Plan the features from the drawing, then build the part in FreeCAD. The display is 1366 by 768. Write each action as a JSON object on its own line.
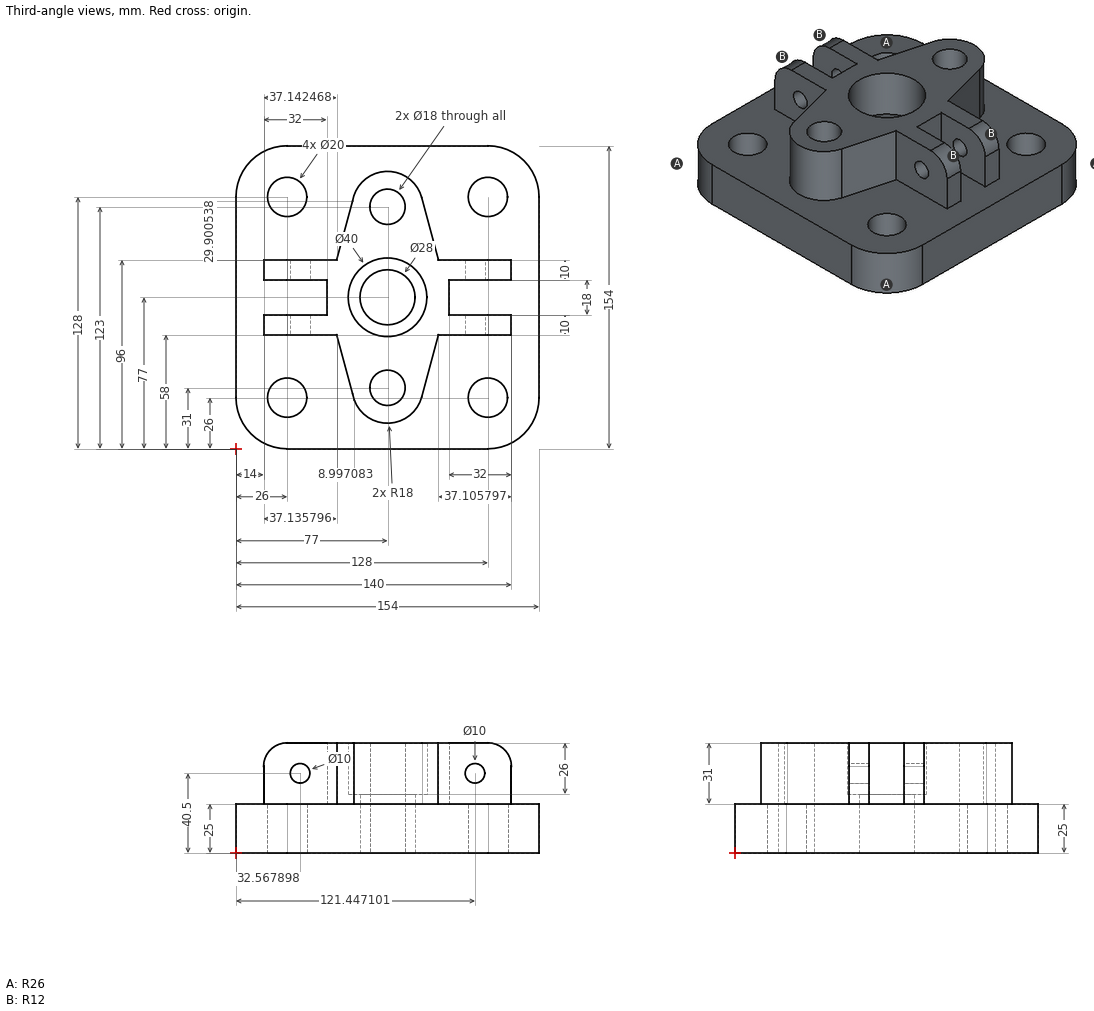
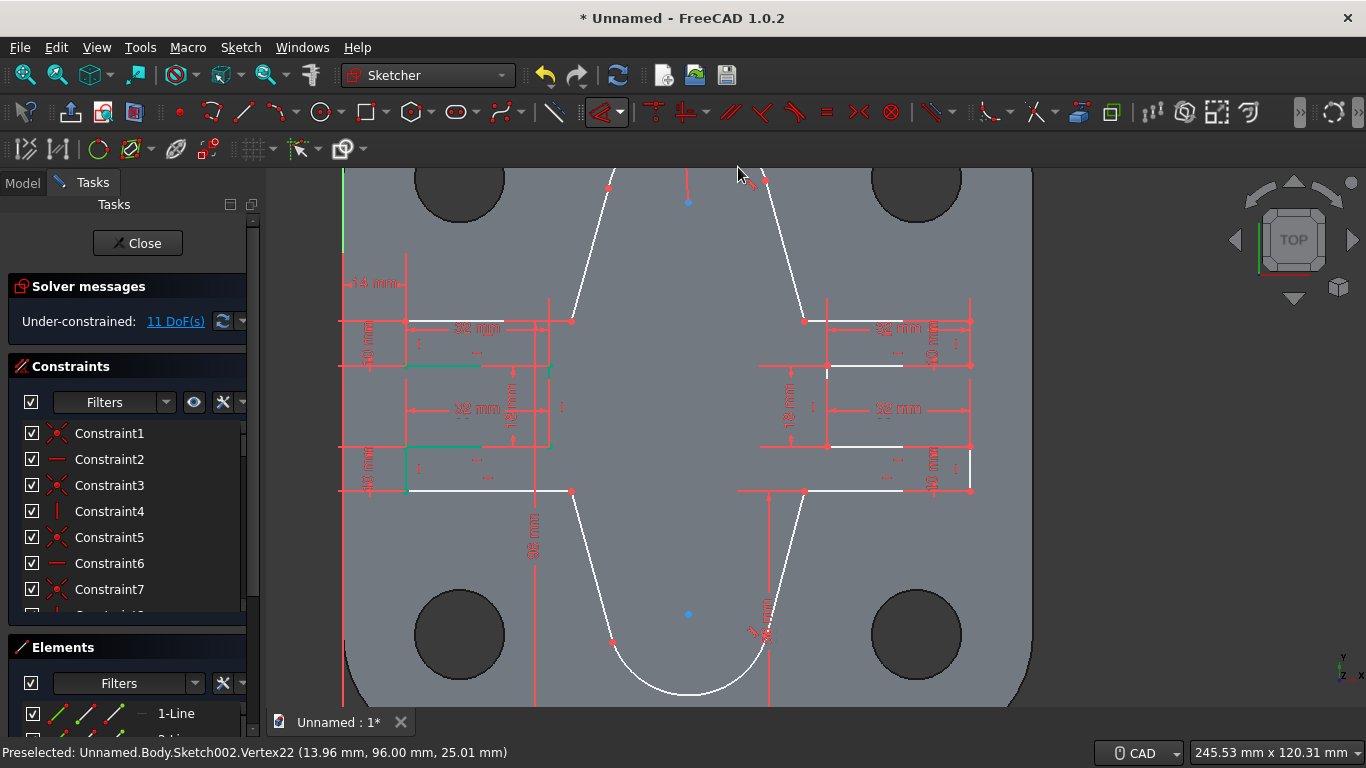
{"action": "left_click", "coordinate": [688, 202]}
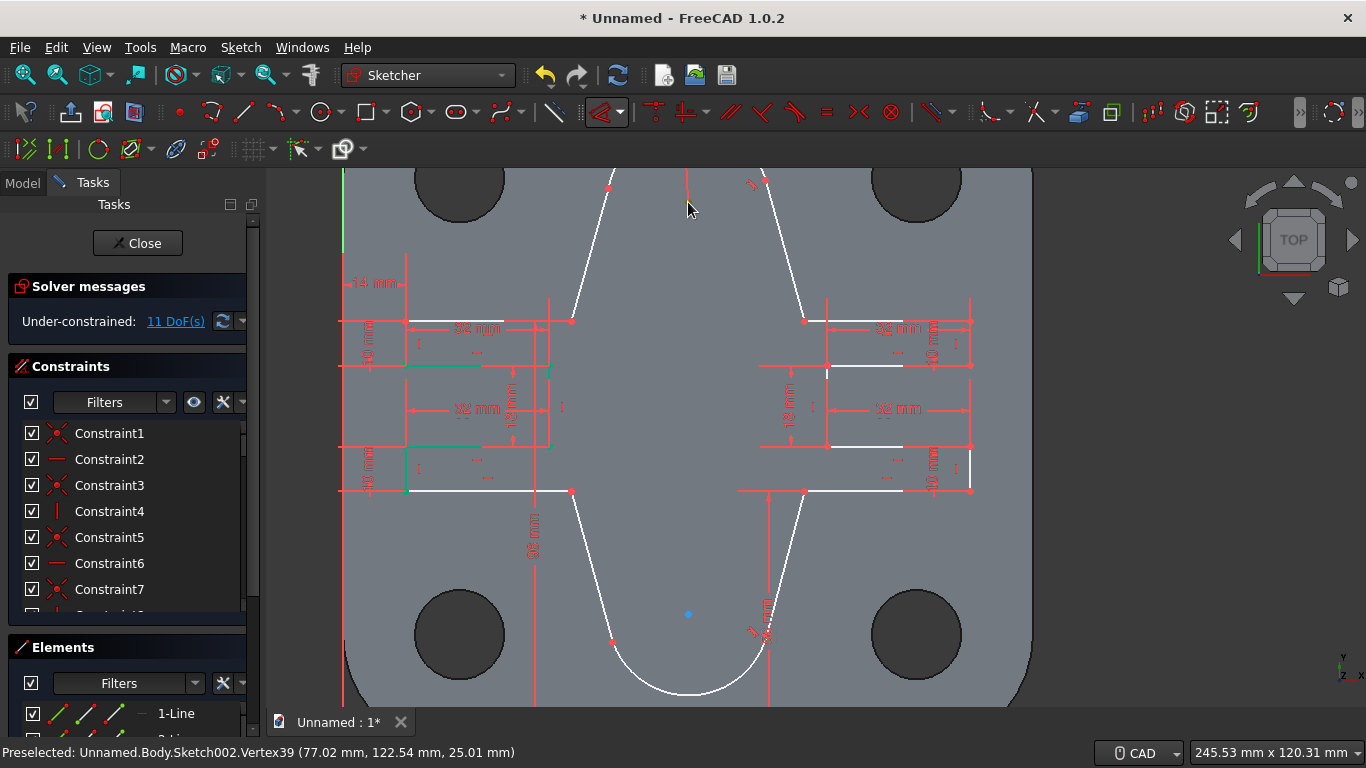
{"action": "left_click", "coordinate": [622, 112]}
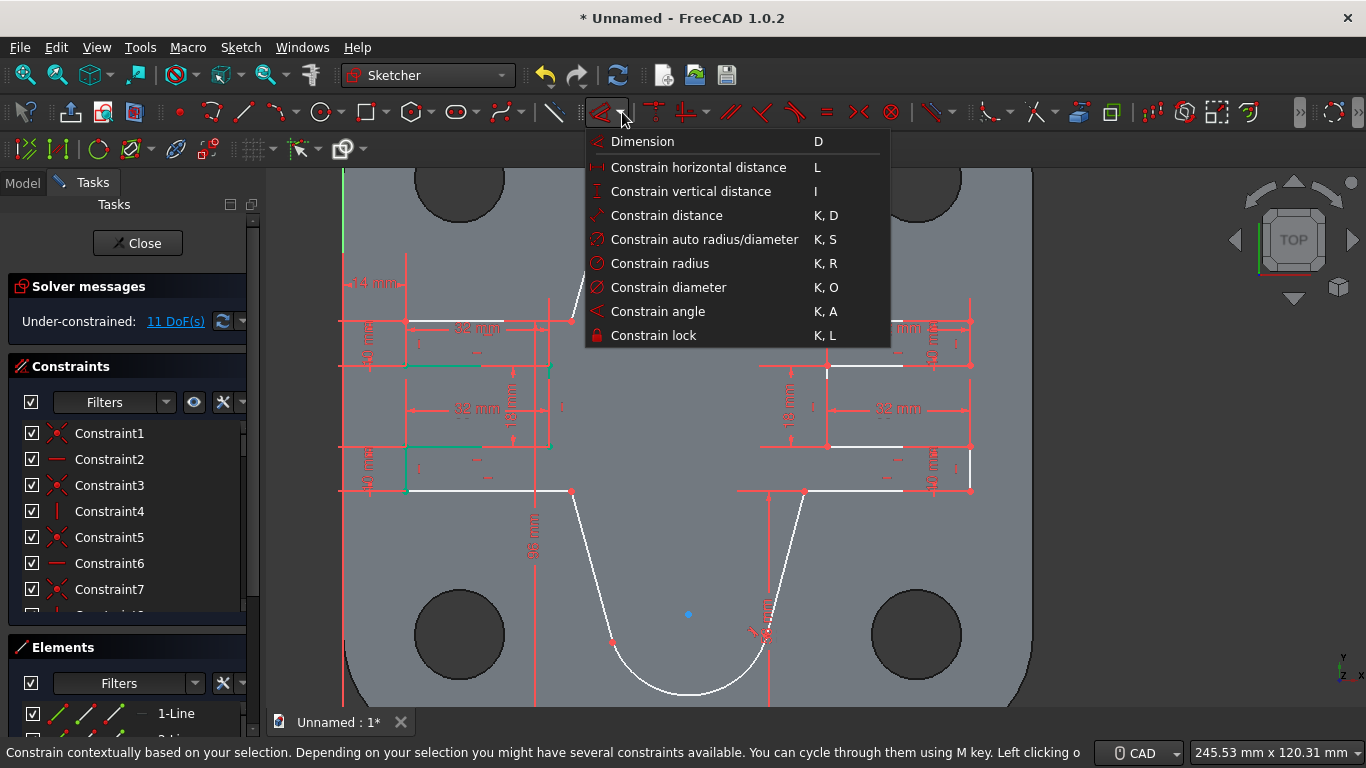
{"action": "left_click", "coordinate": [738, 167]}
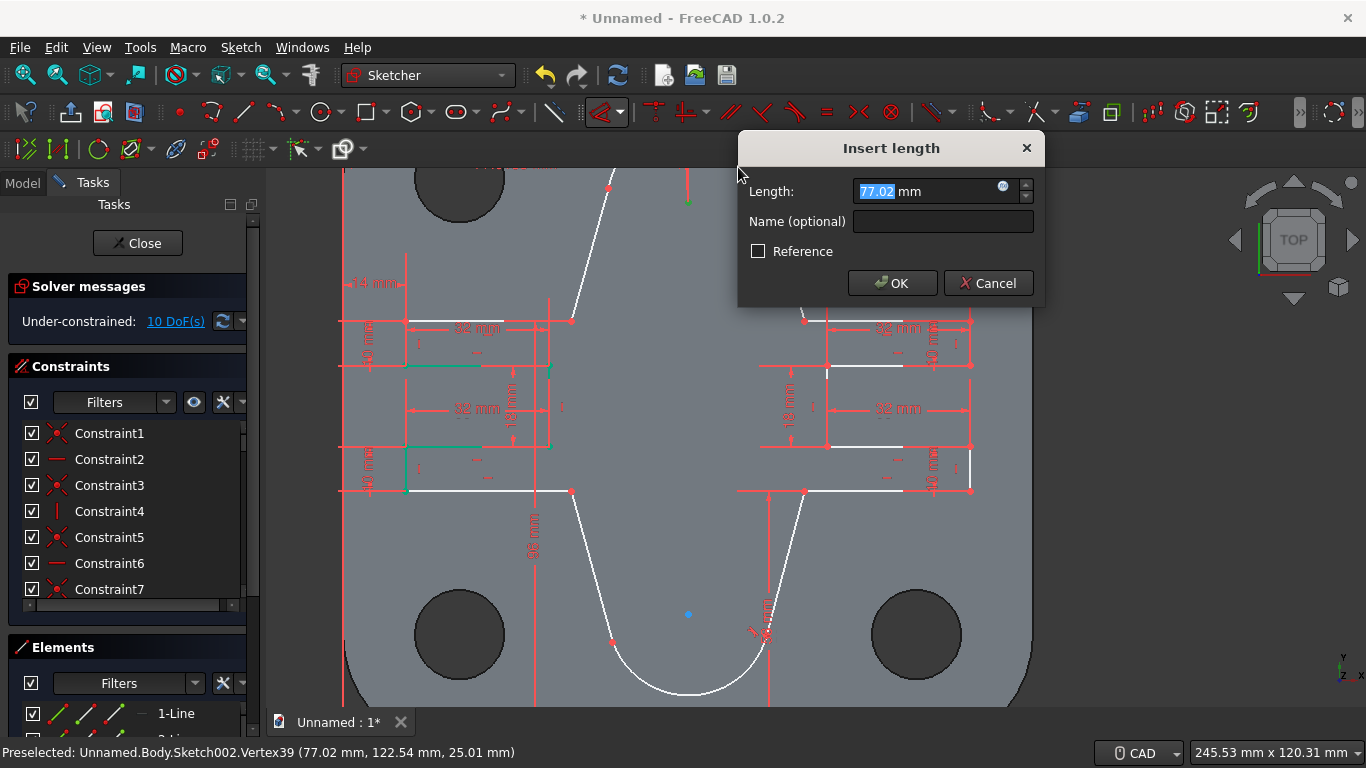
{"action": "type", "text": "77"}
{"action": "key", "text": "Return"}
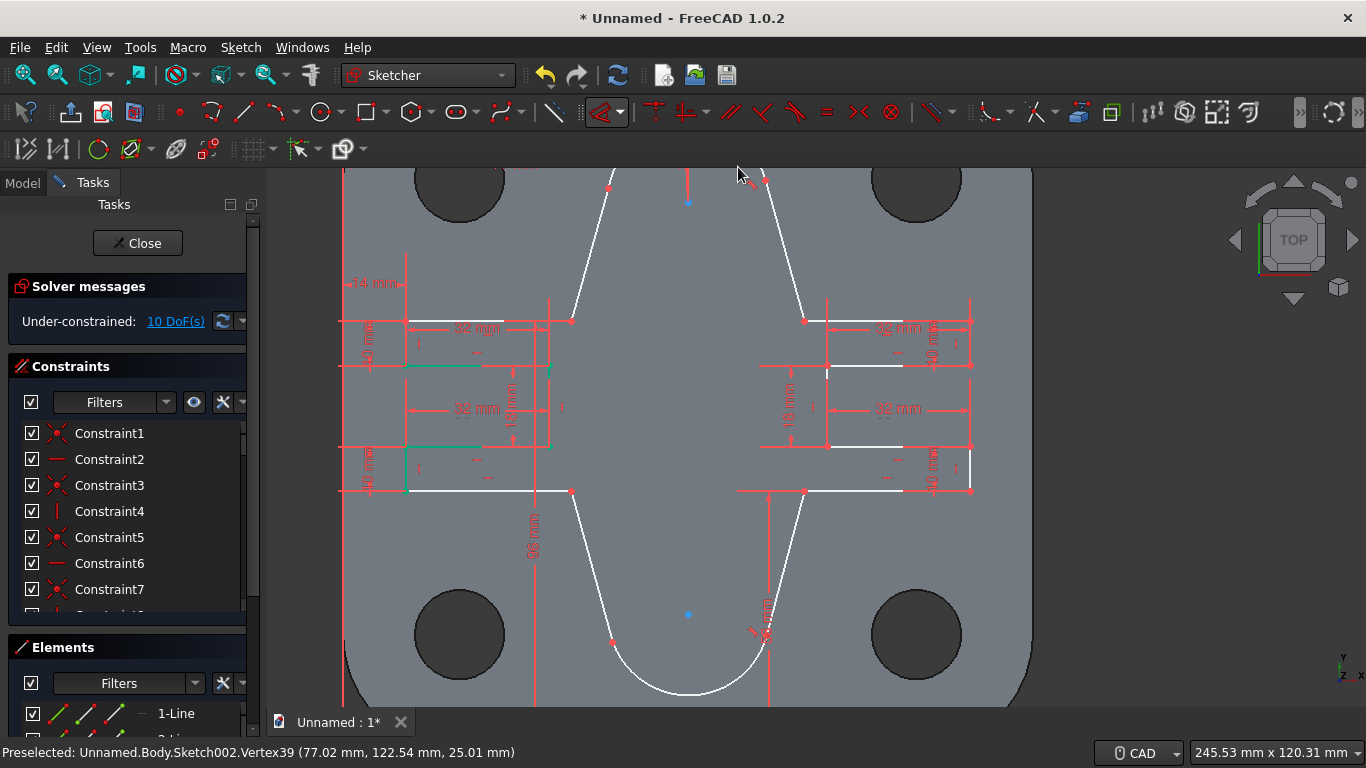
{"action": "left_click", "coordinate": [689, 615]}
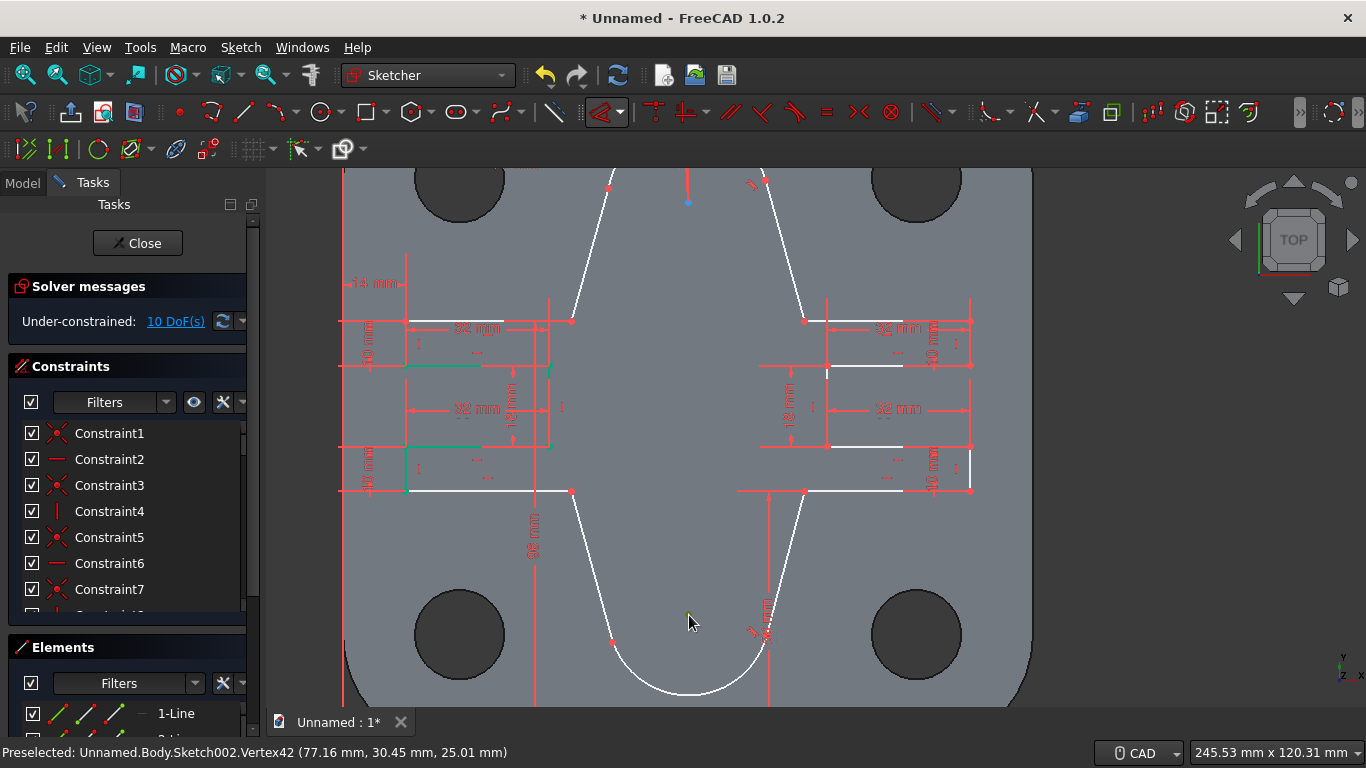
{"action": "left_click", "coordinate": [622, 112]}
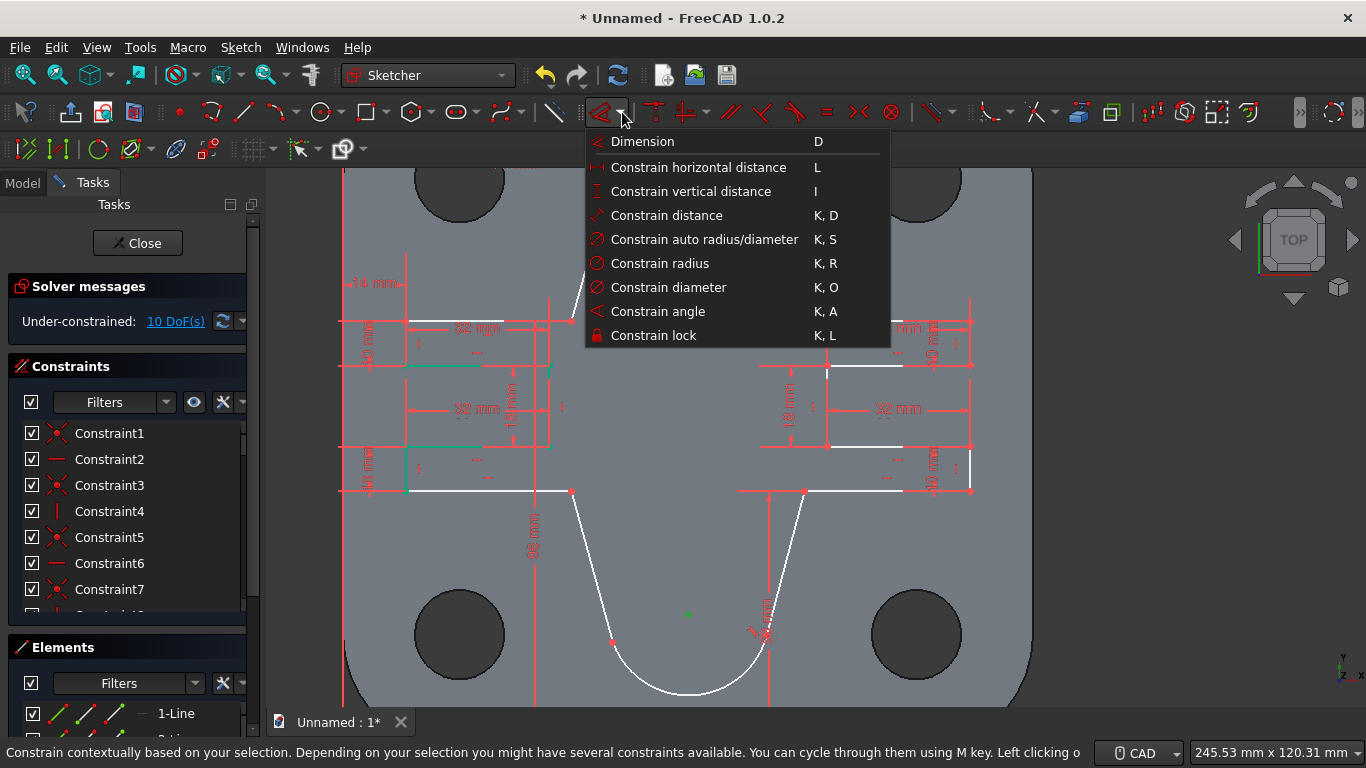
{"action": "left_click", "coordinate": [738, 167]}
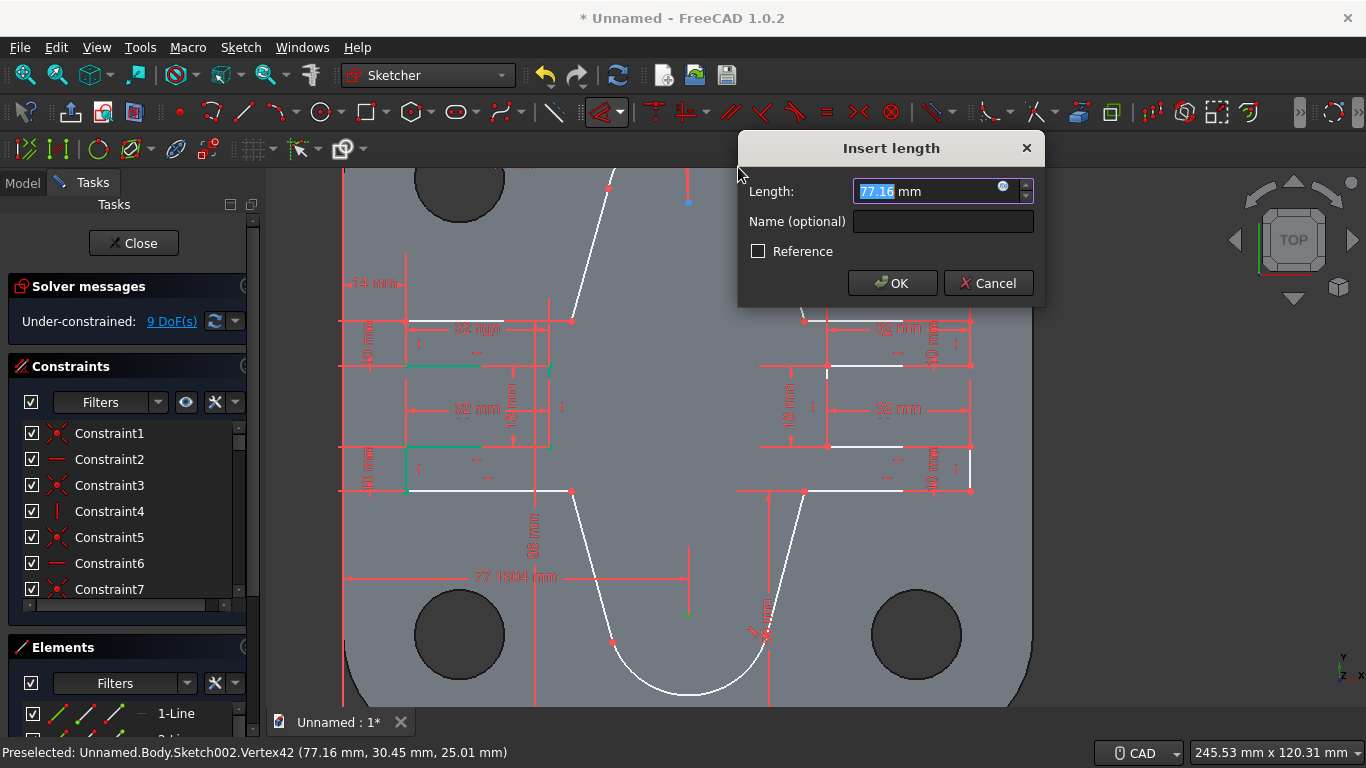
{"action": "type", "text": "77"}
{"action": "key", "text": "Return"}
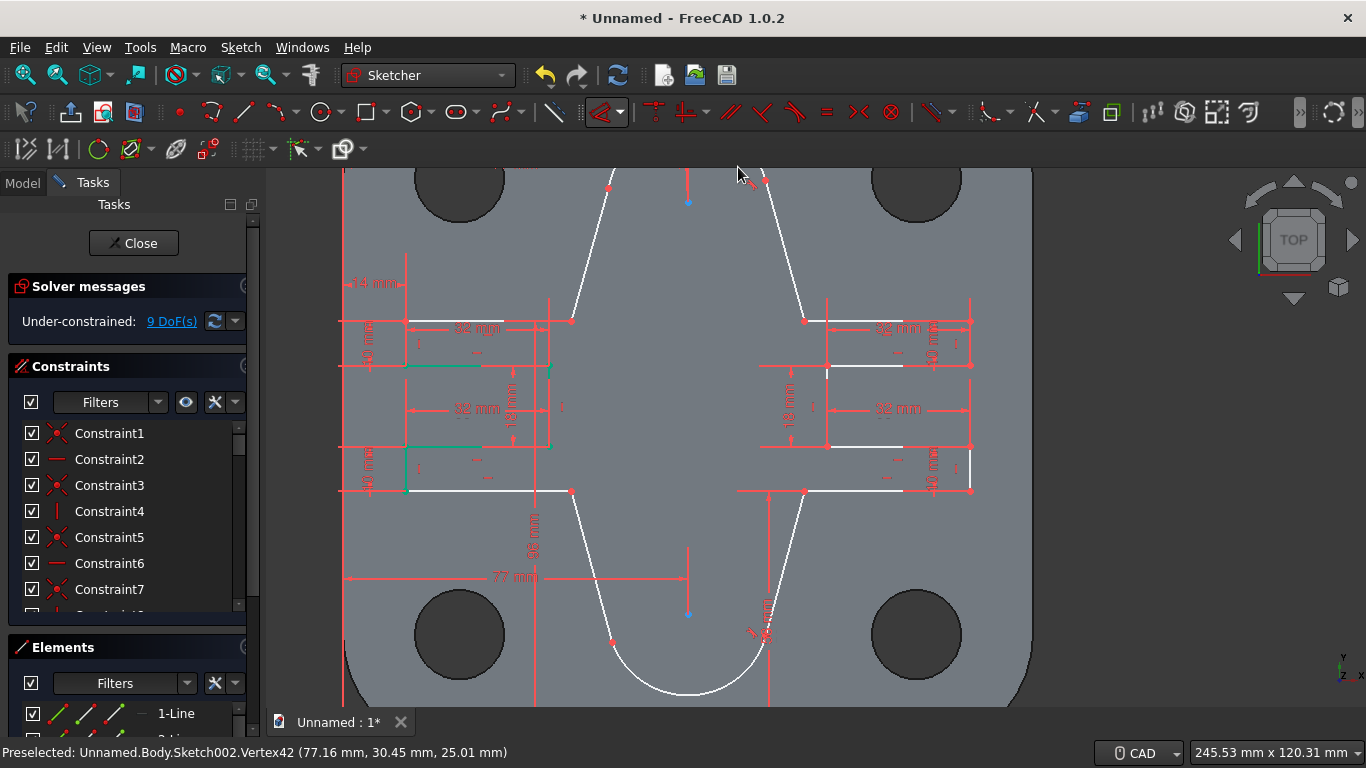
{"action": "left_click", "coordinate": [688, 615]}